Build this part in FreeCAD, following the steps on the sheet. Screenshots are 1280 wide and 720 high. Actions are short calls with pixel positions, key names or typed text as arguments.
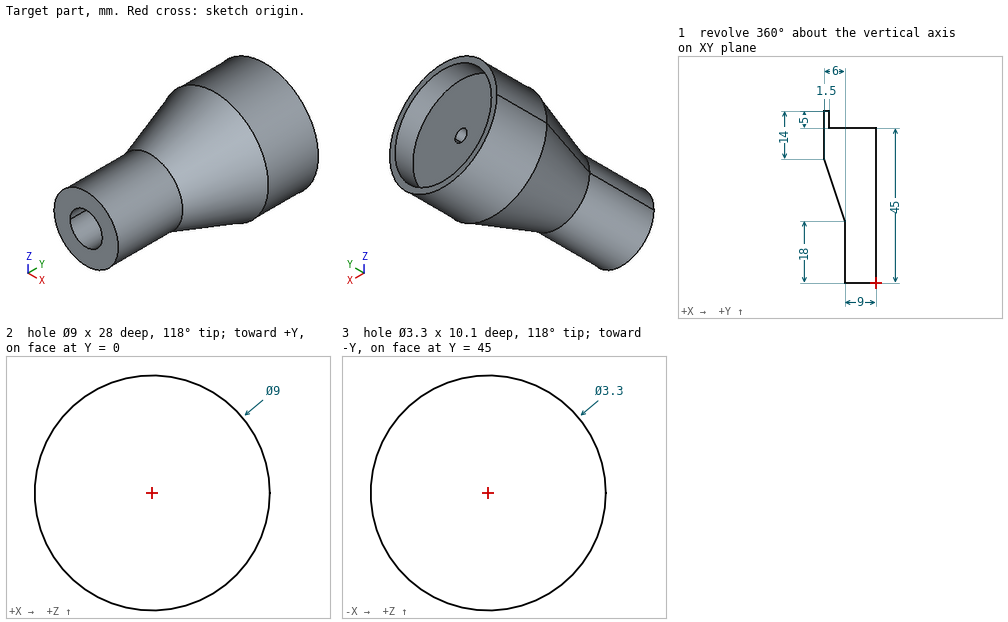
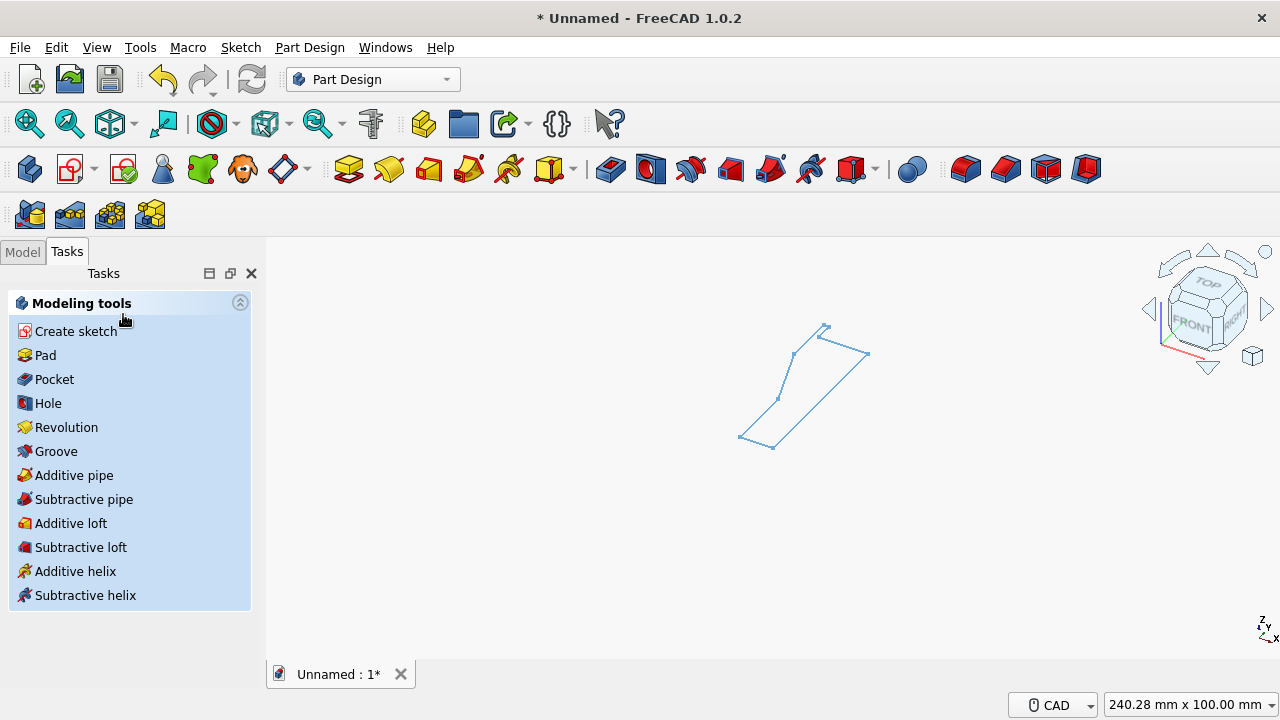
click(390, 170)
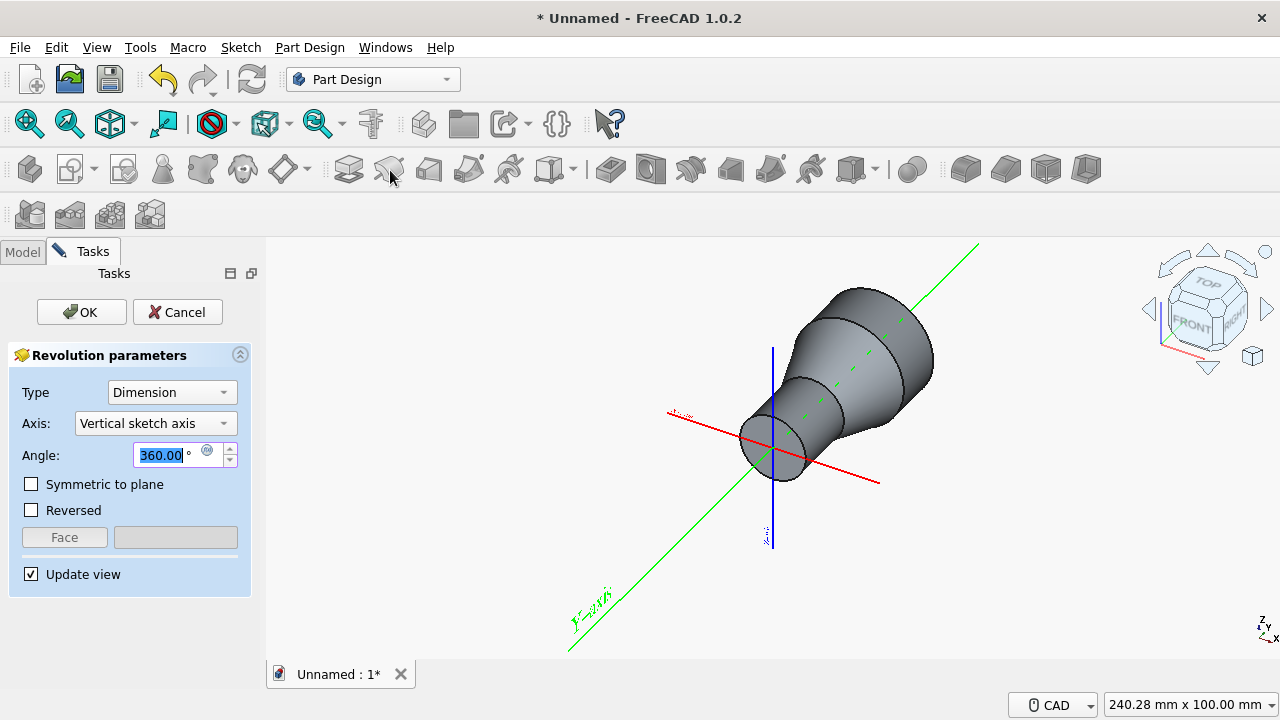
click(82, 312)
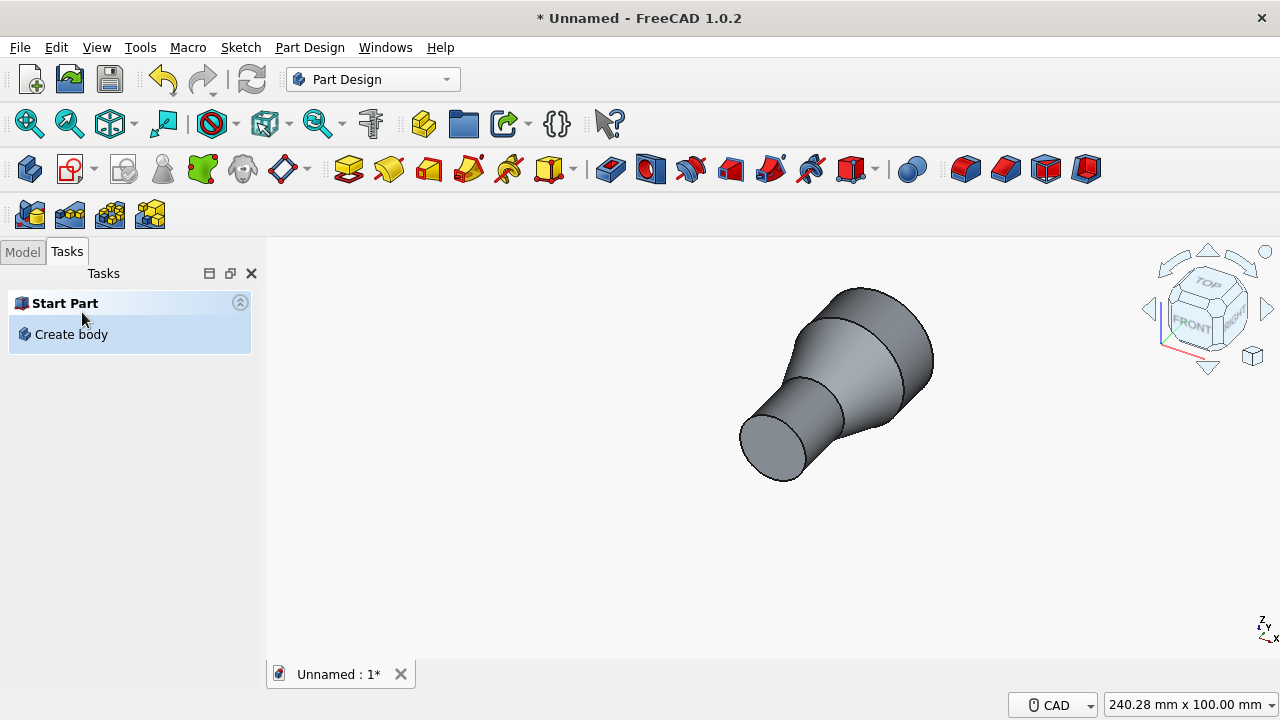
click(773, 447)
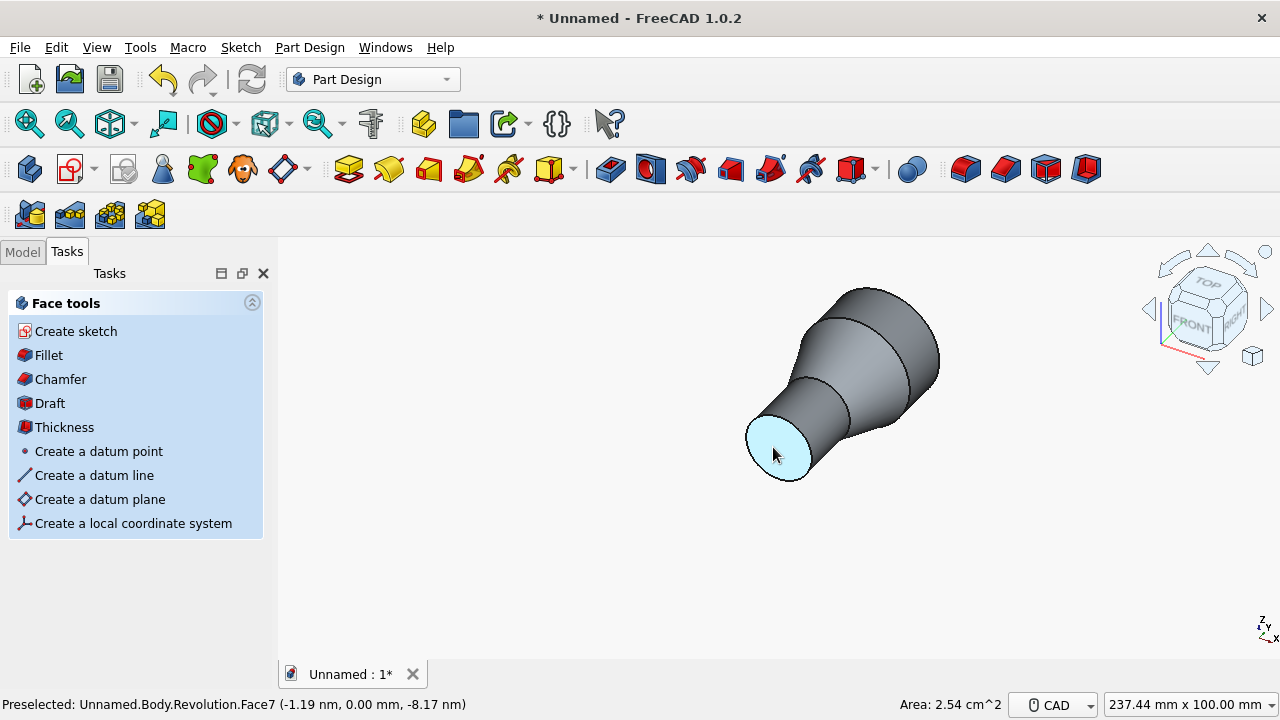
click(70, 170)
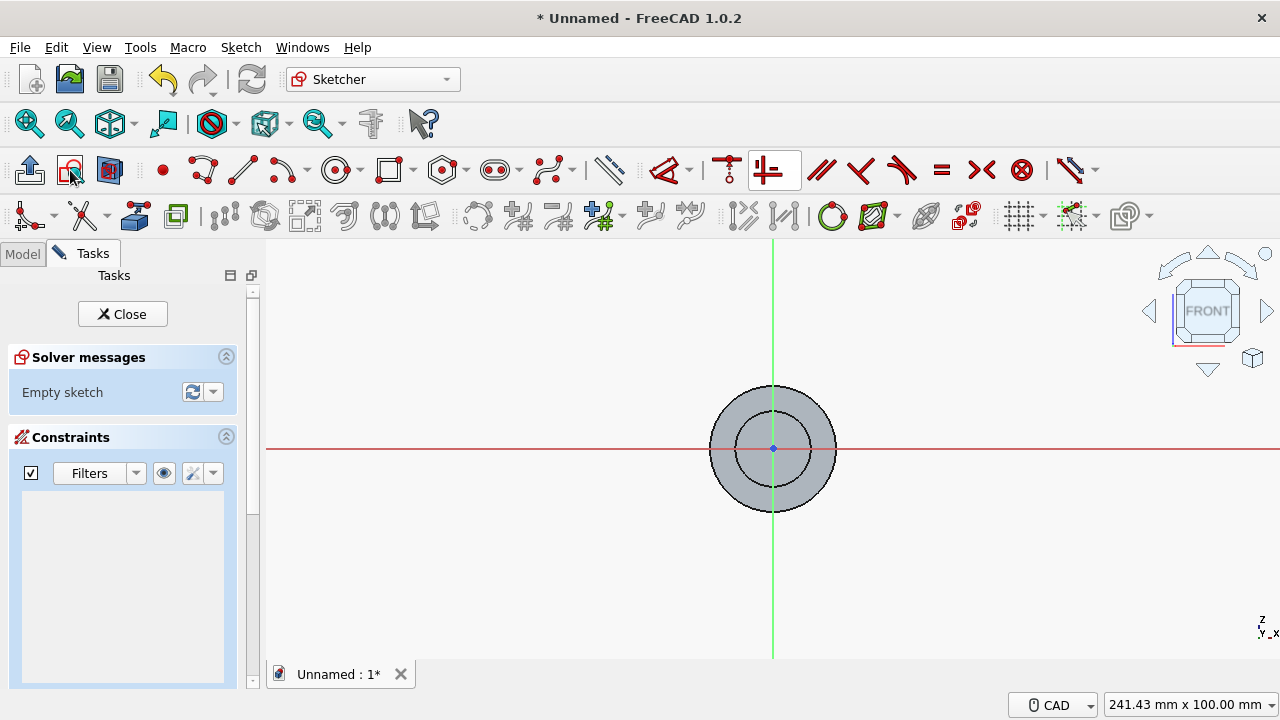
scroll(784, 449, up, 10)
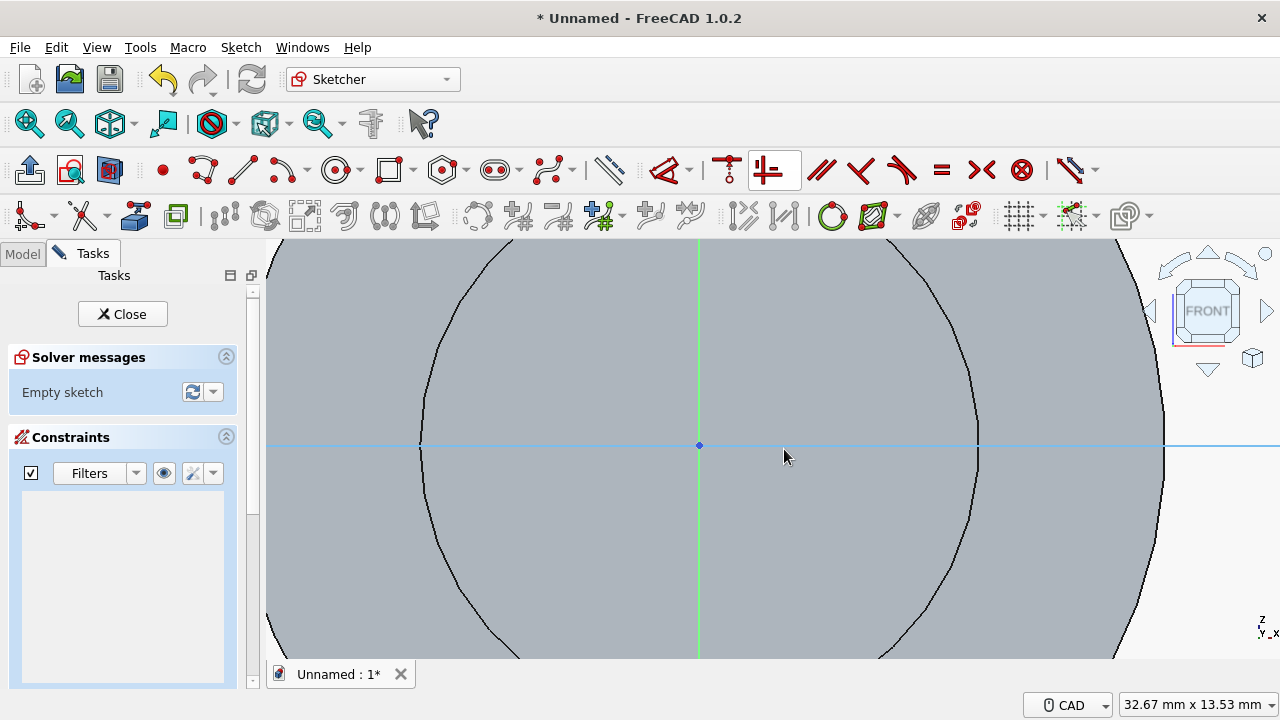
click(336, 170)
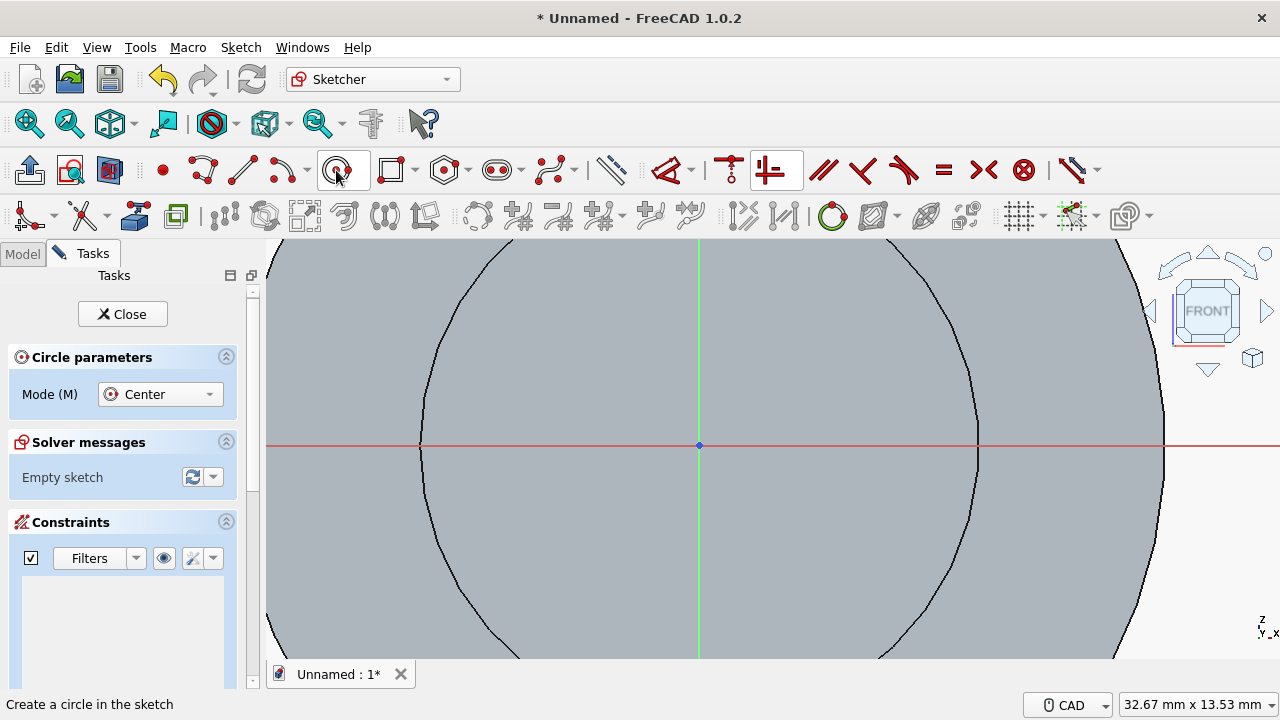
click(699, 446)
move(798, 347)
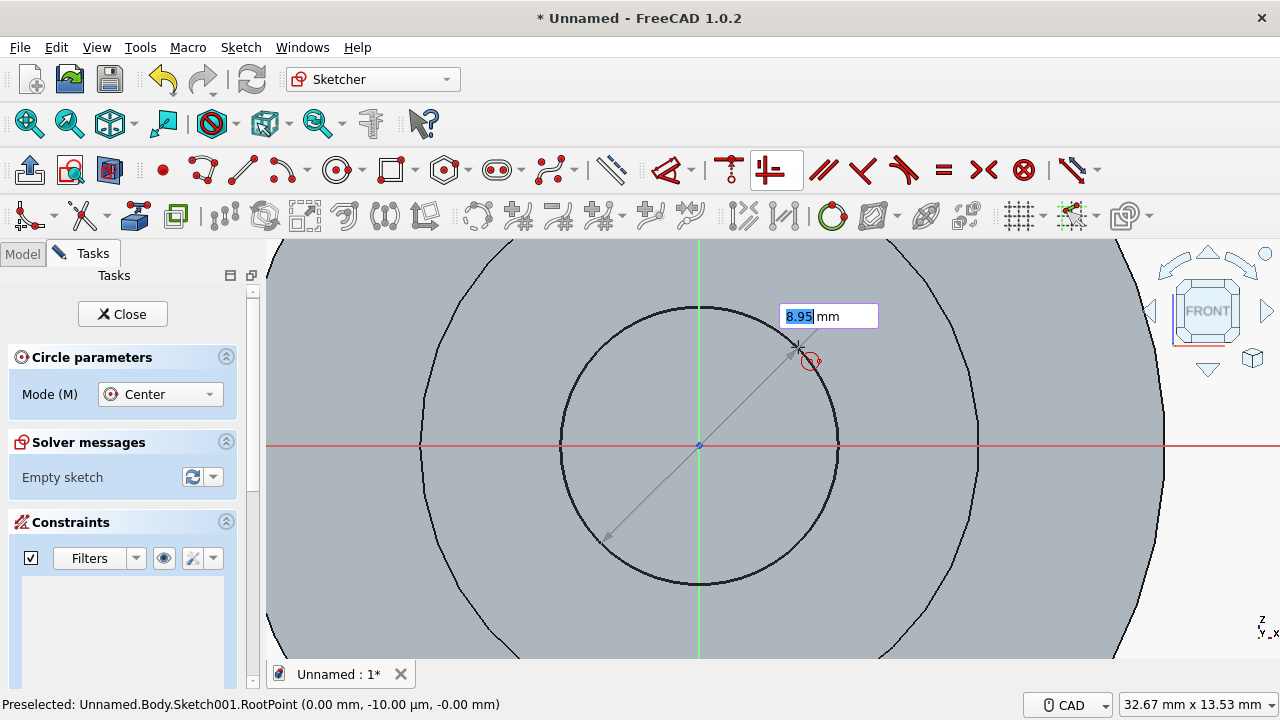
text(9)
key(Return)
key(Escape)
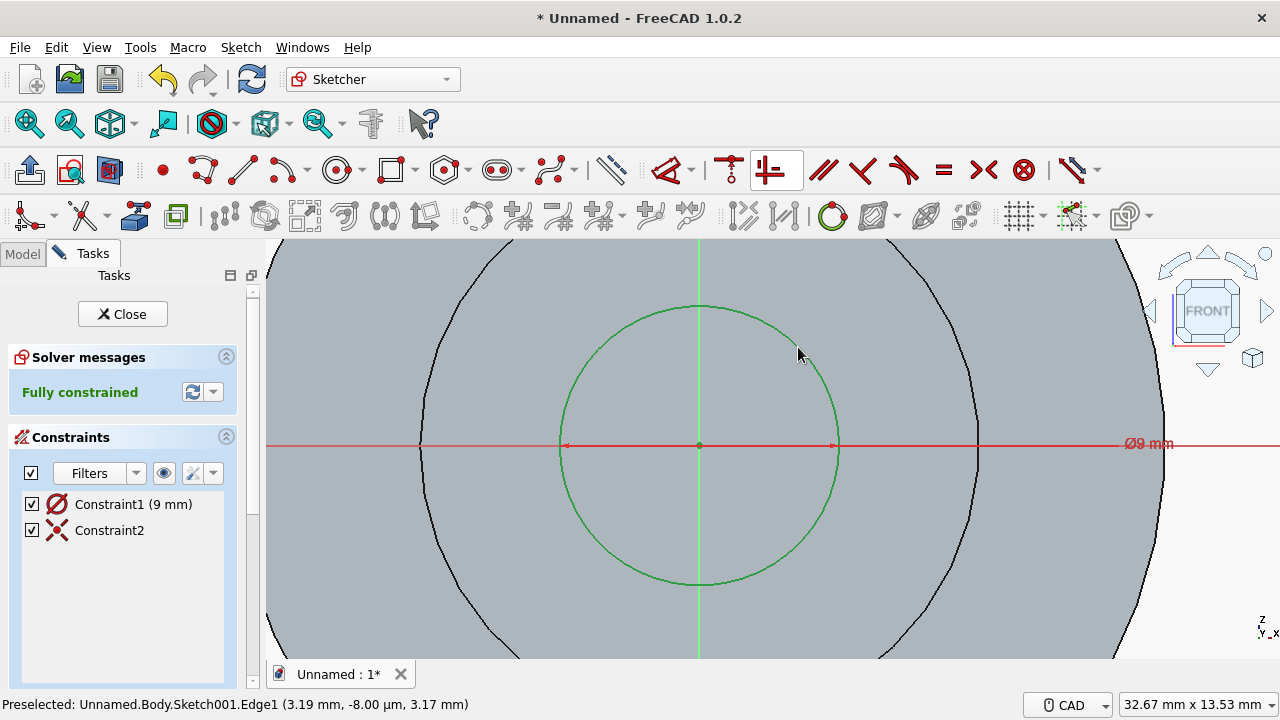
click(123, 314)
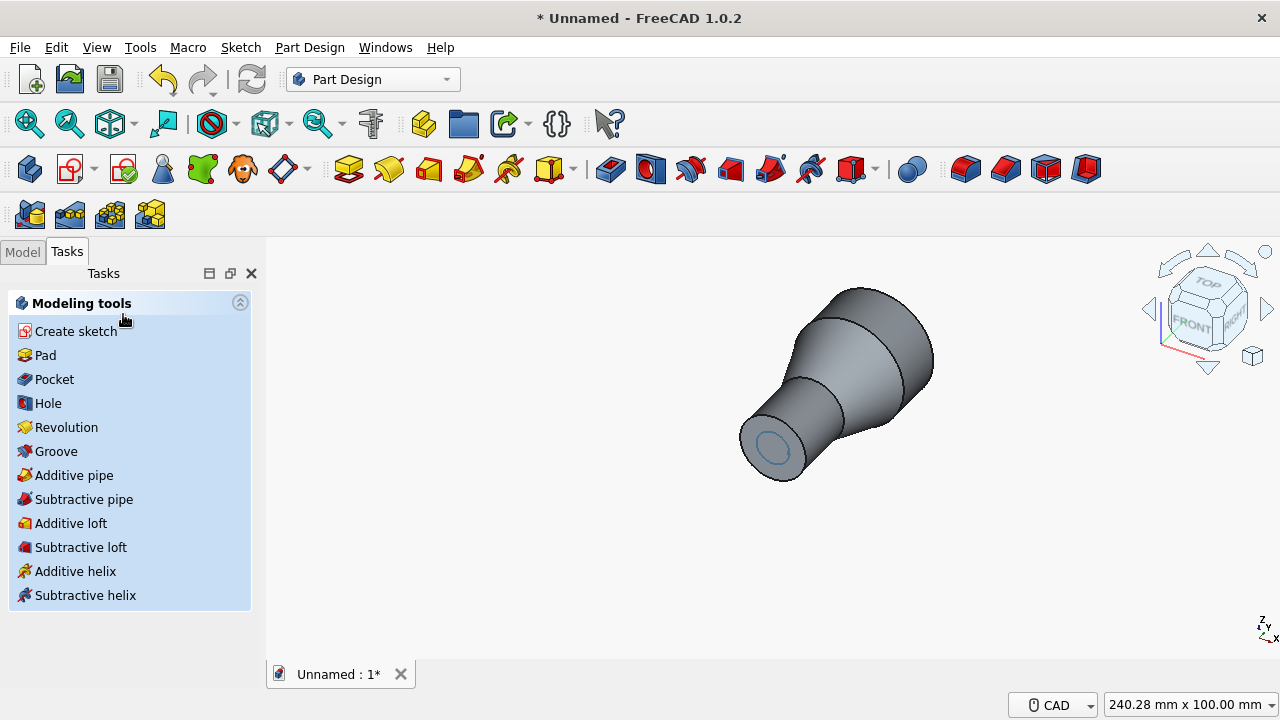
click(652, 170)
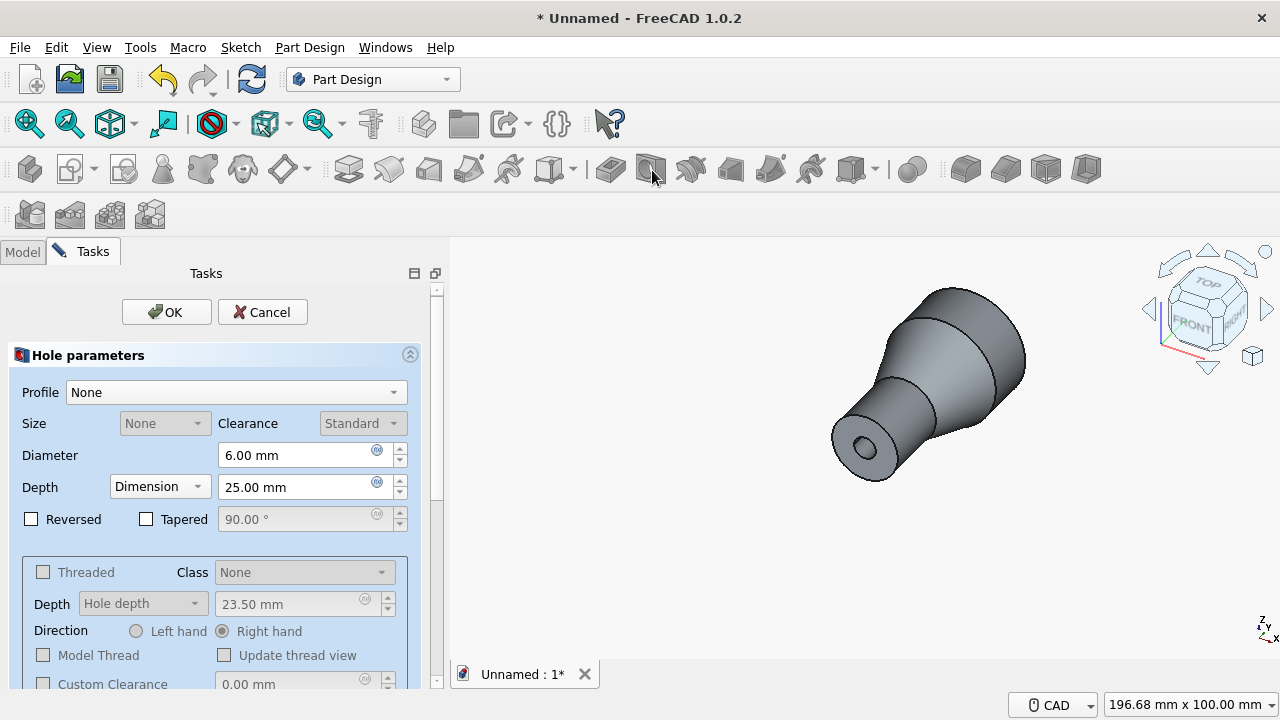
triple_click(305, 455)